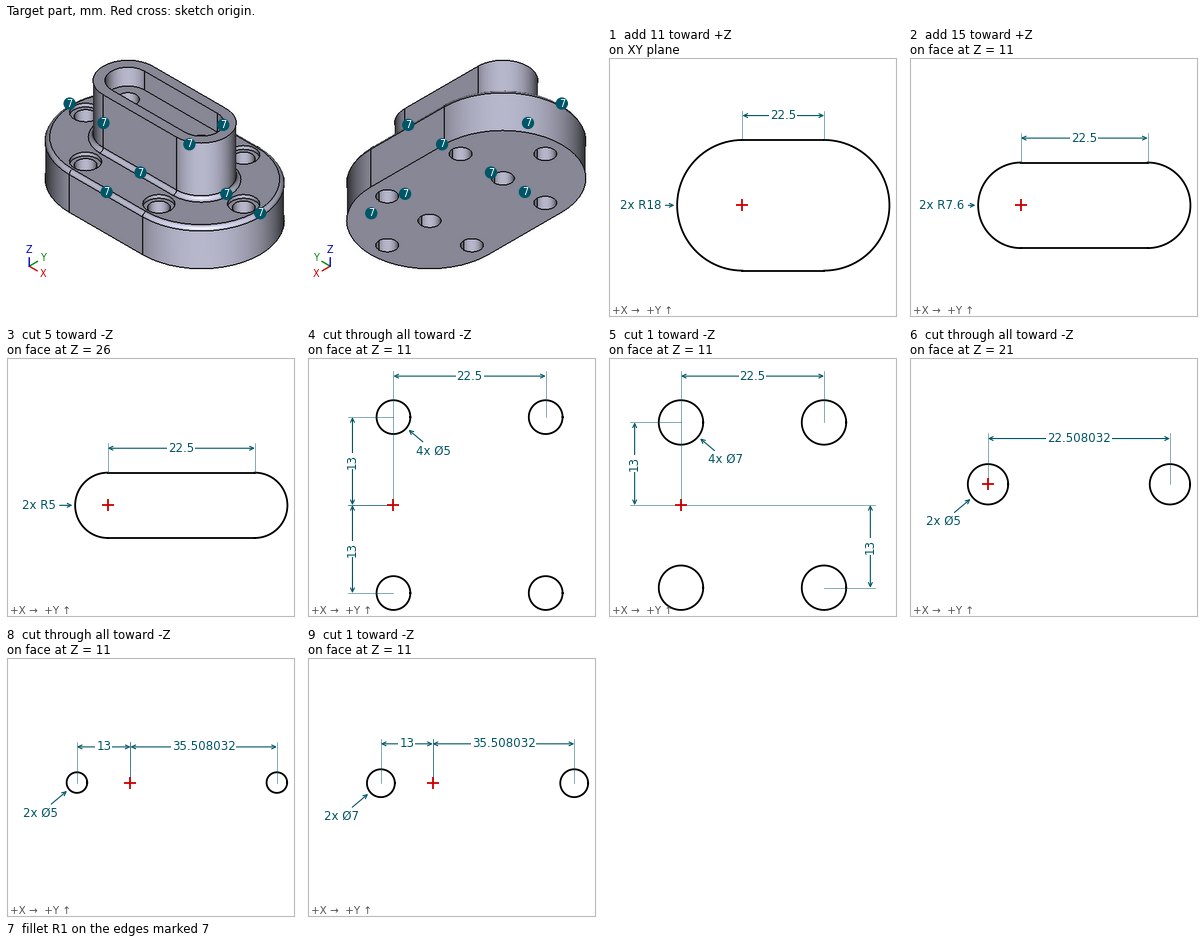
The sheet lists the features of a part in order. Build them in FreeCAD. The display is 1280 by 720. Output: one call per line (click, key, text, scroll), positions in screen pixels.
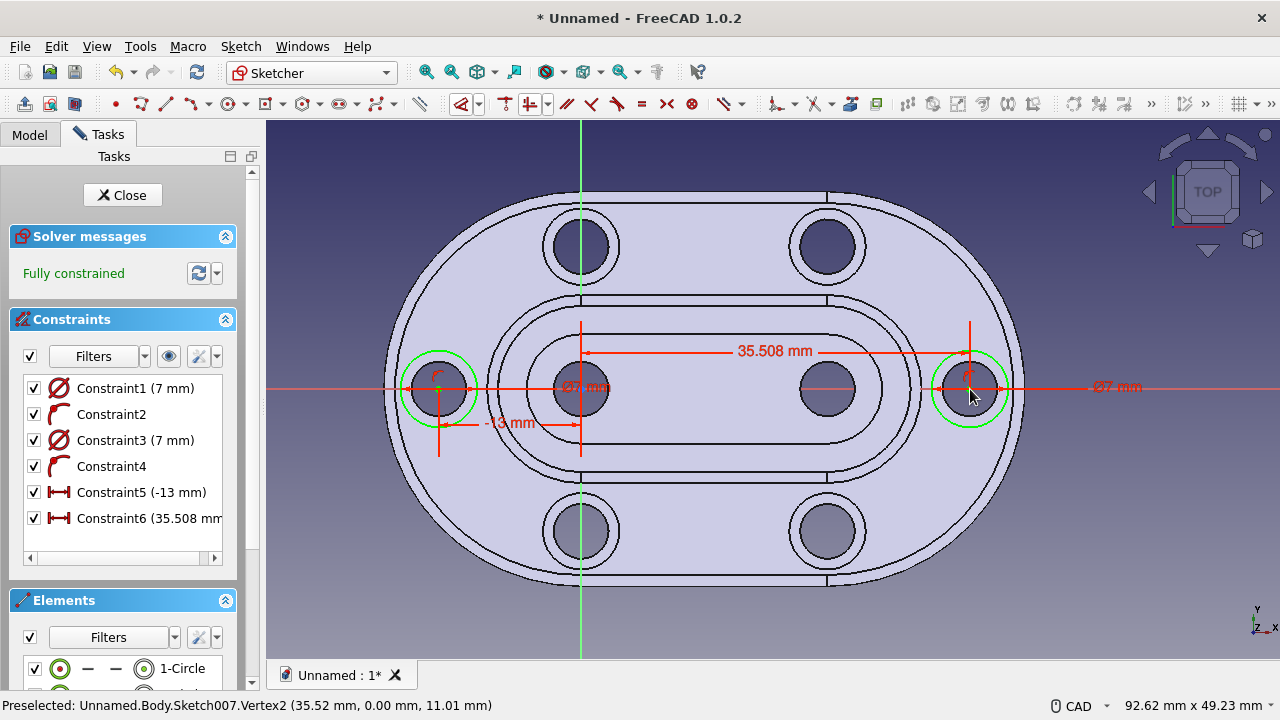
click(123, 195)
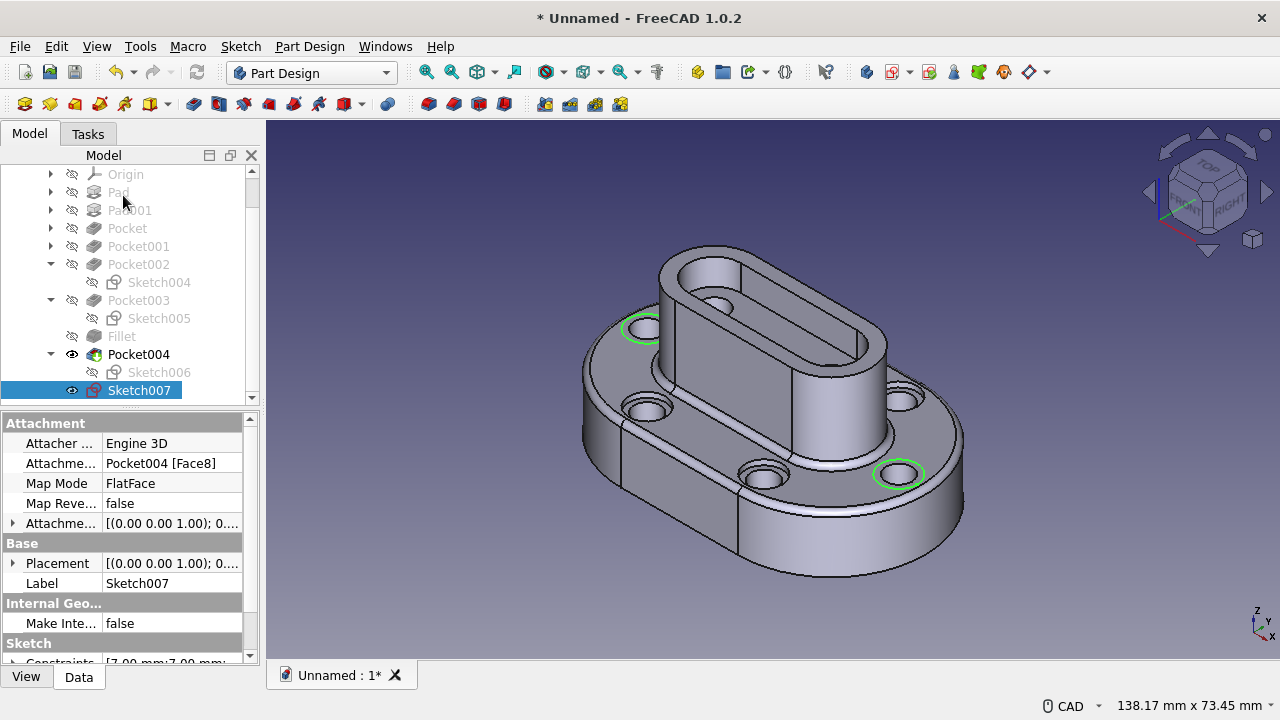
click(194, 104)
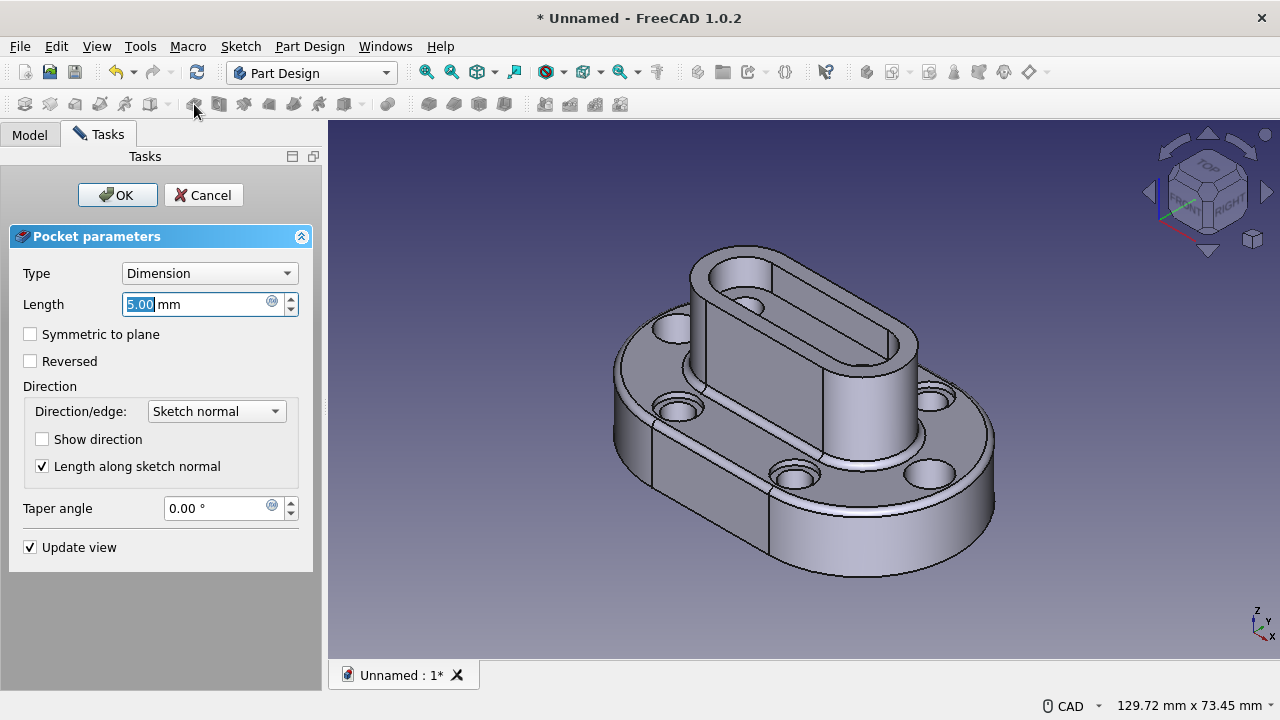
text(1)
key(Tab)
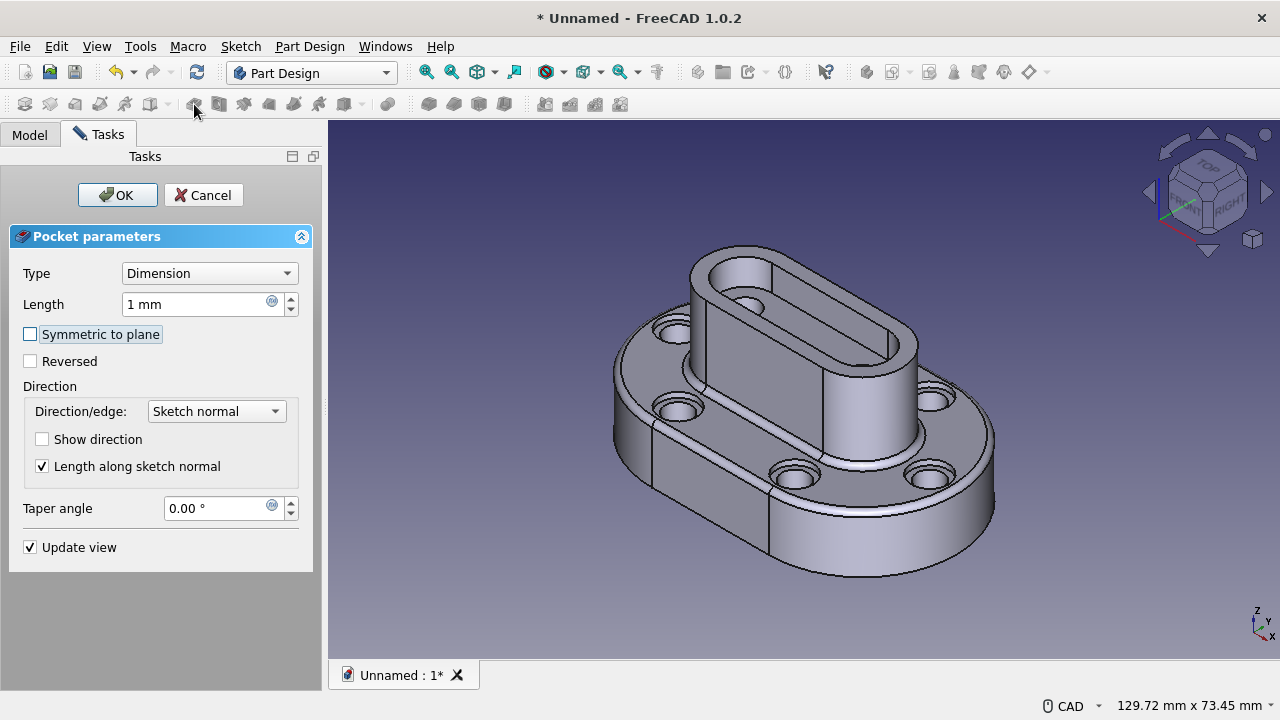
click(118, 195)